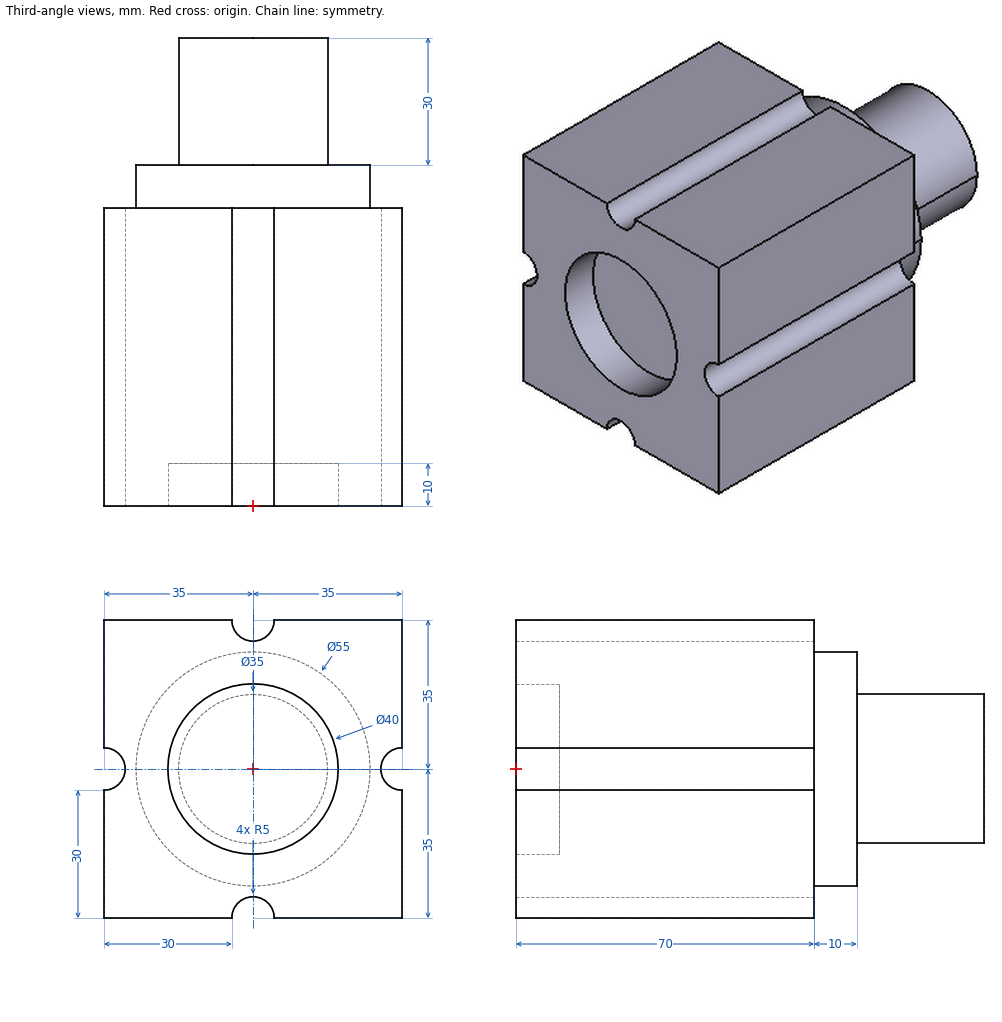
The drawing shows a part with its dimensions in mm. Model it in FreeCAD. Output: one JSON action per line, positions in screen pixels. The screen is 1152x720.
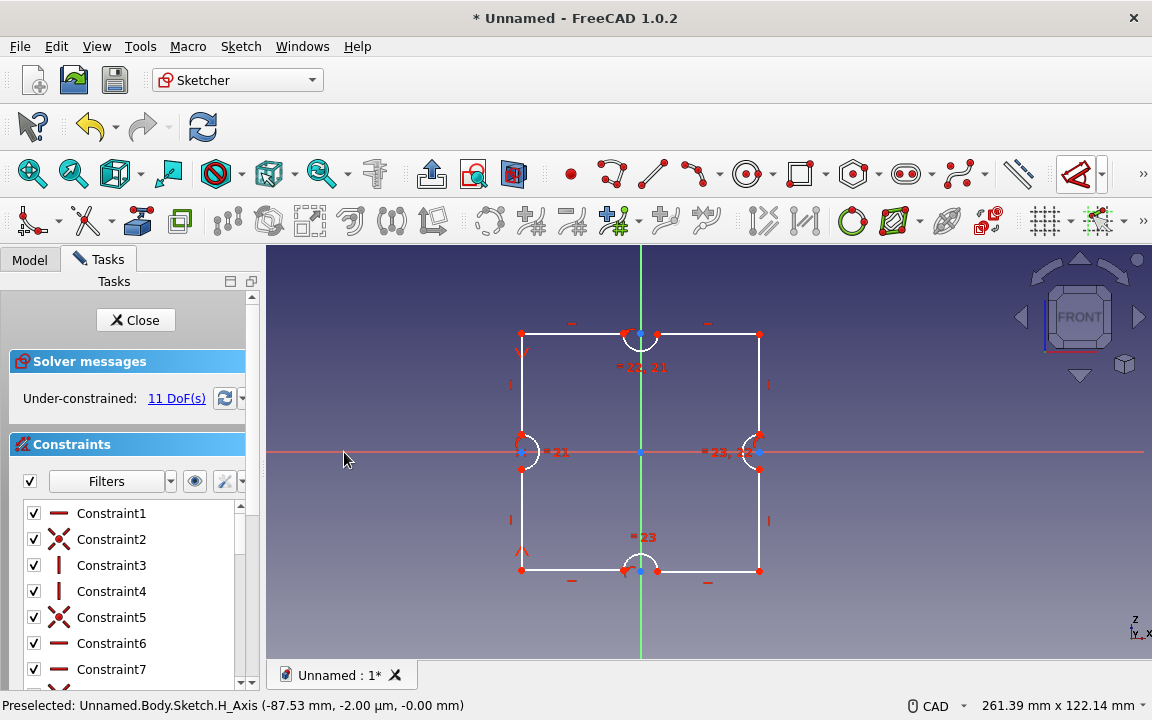
{"action": "left_click", "coordinate": [522, 334]}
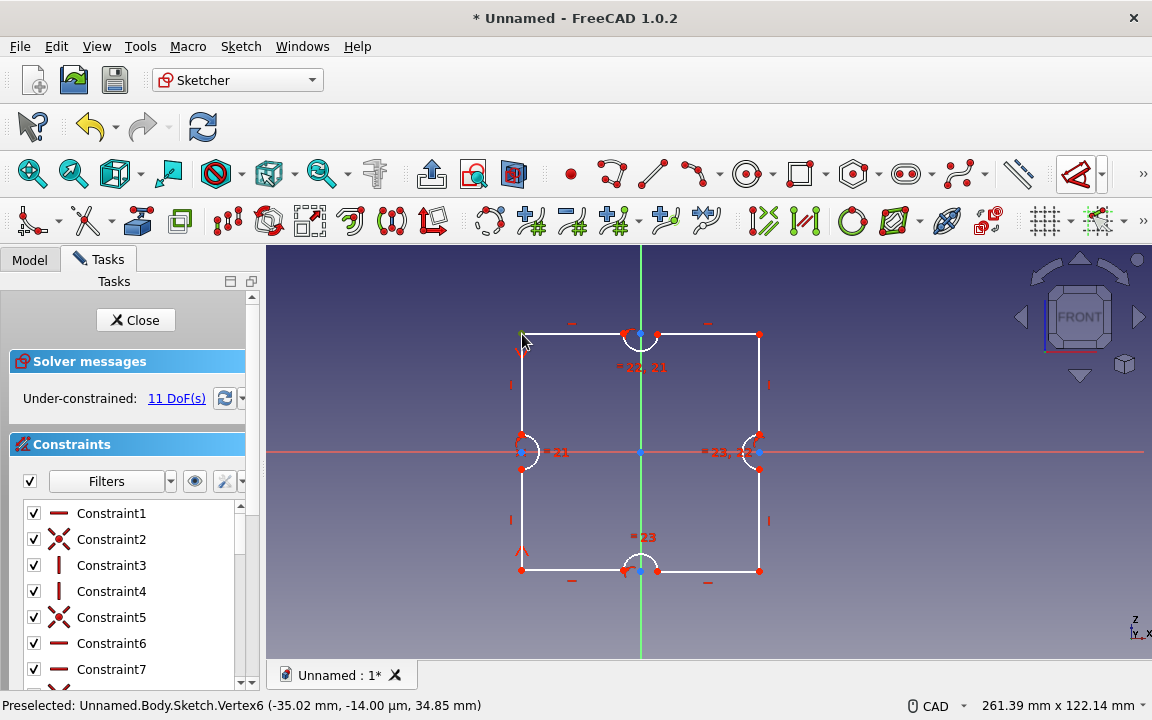
{"action": "left_click", "coordinate": [759, 334]}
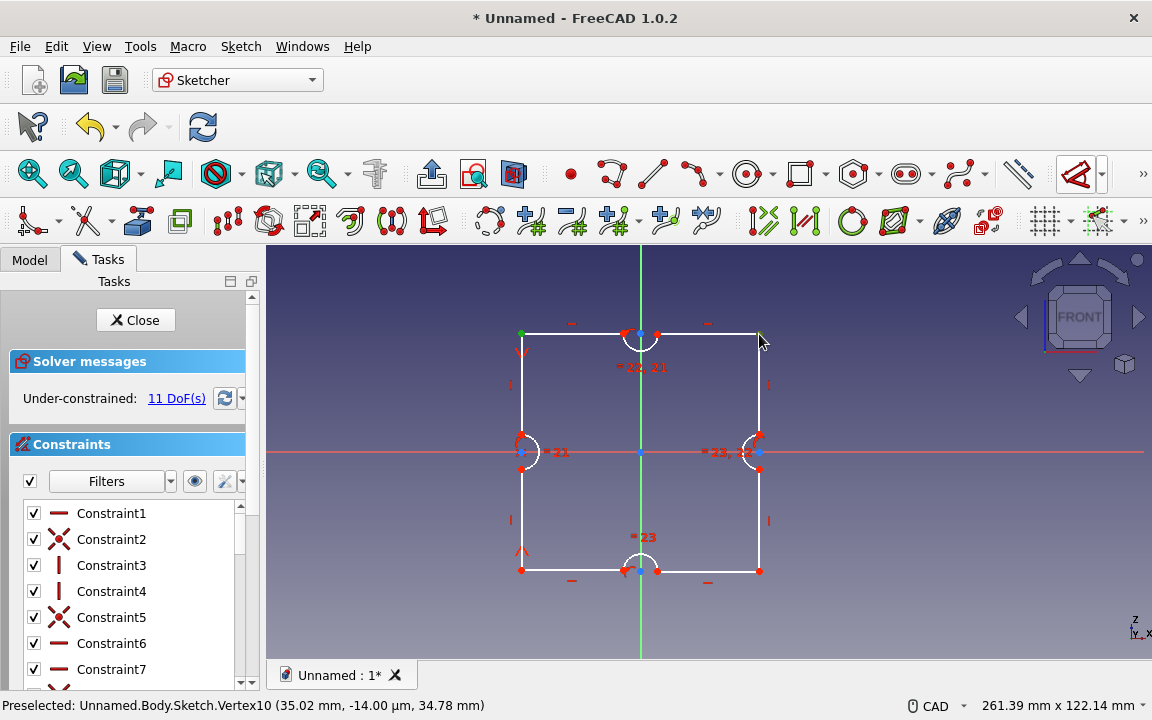
{"action": "left_click", "coordinate": [641, 605]}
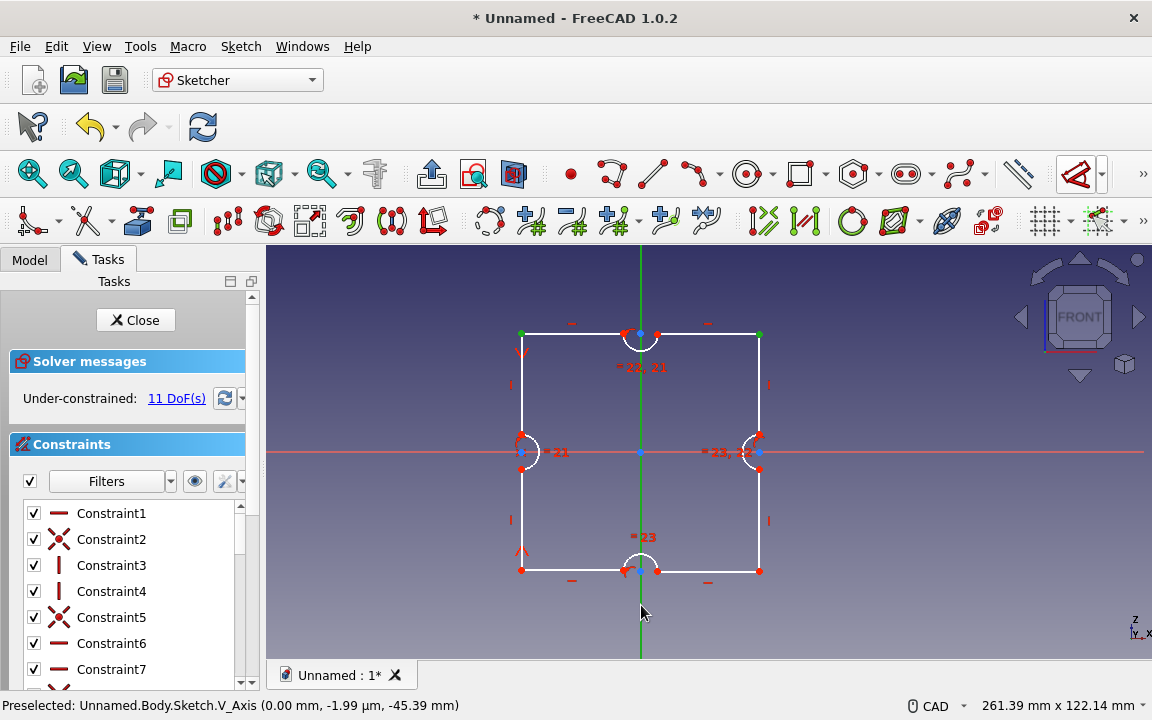
{"action": "key", "text": "s"}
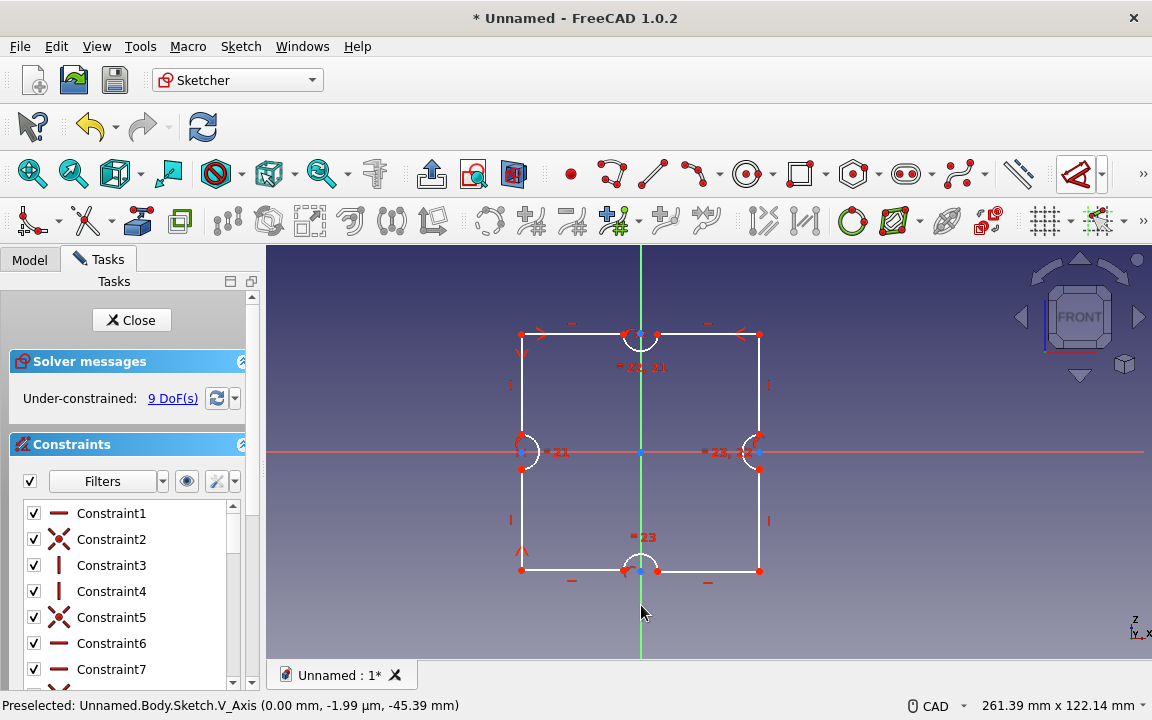
{"action": "left_click", "coordinate": [522, 570]}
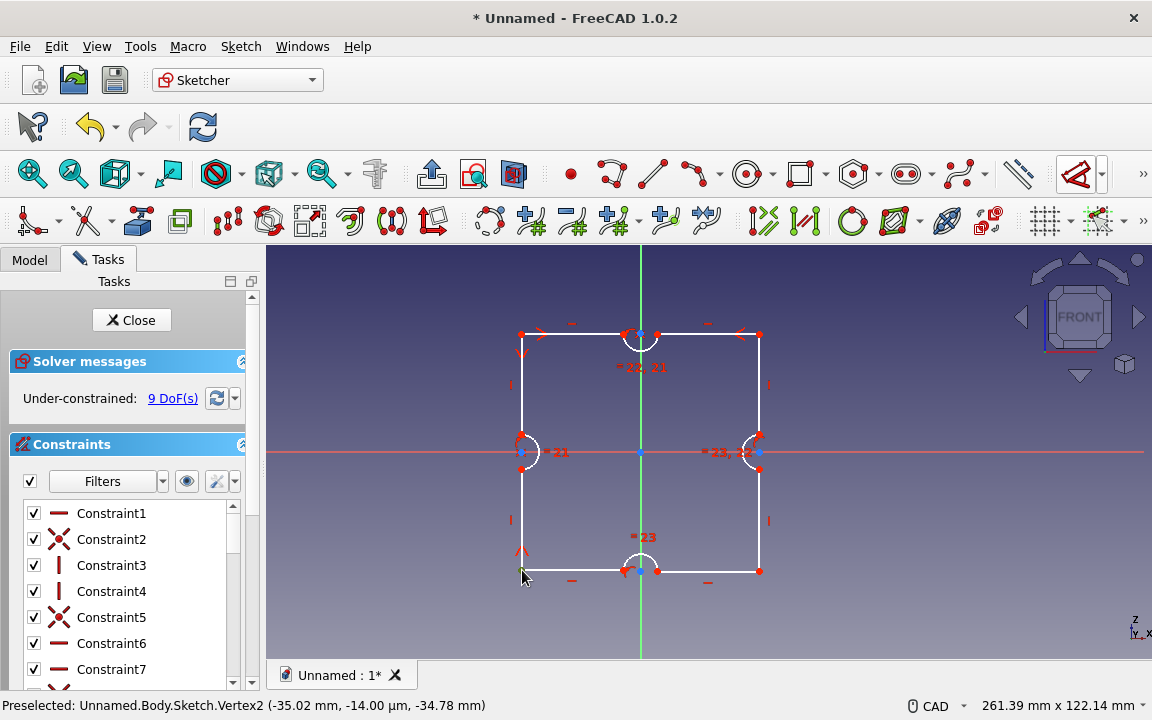
{"action": "left_click", "coordinate": [759, 572]}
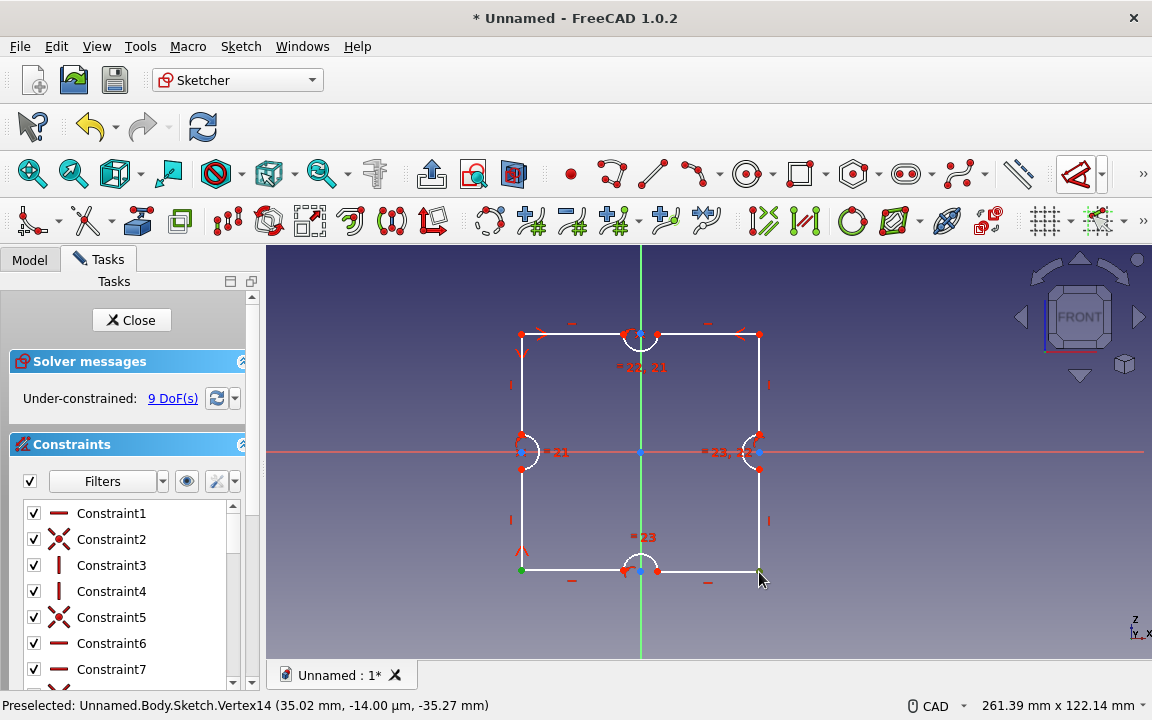
{"action": "left_click", "coordinate": [641, 605]}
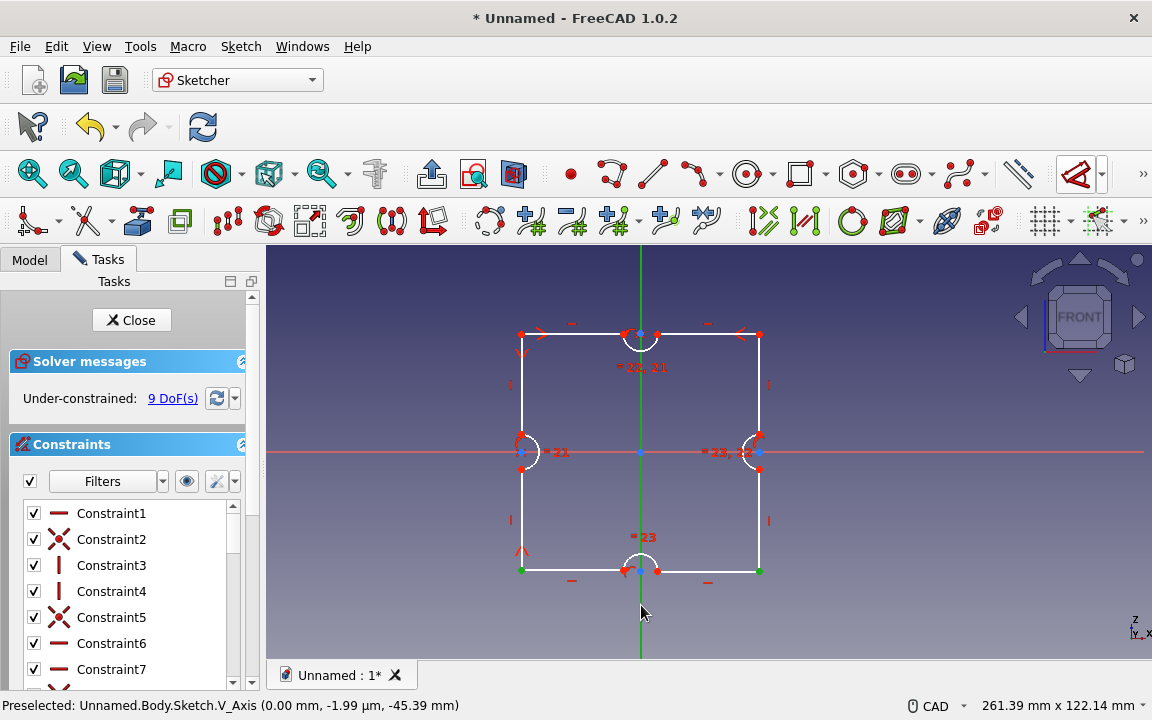
{"action": "key", "text": "s"}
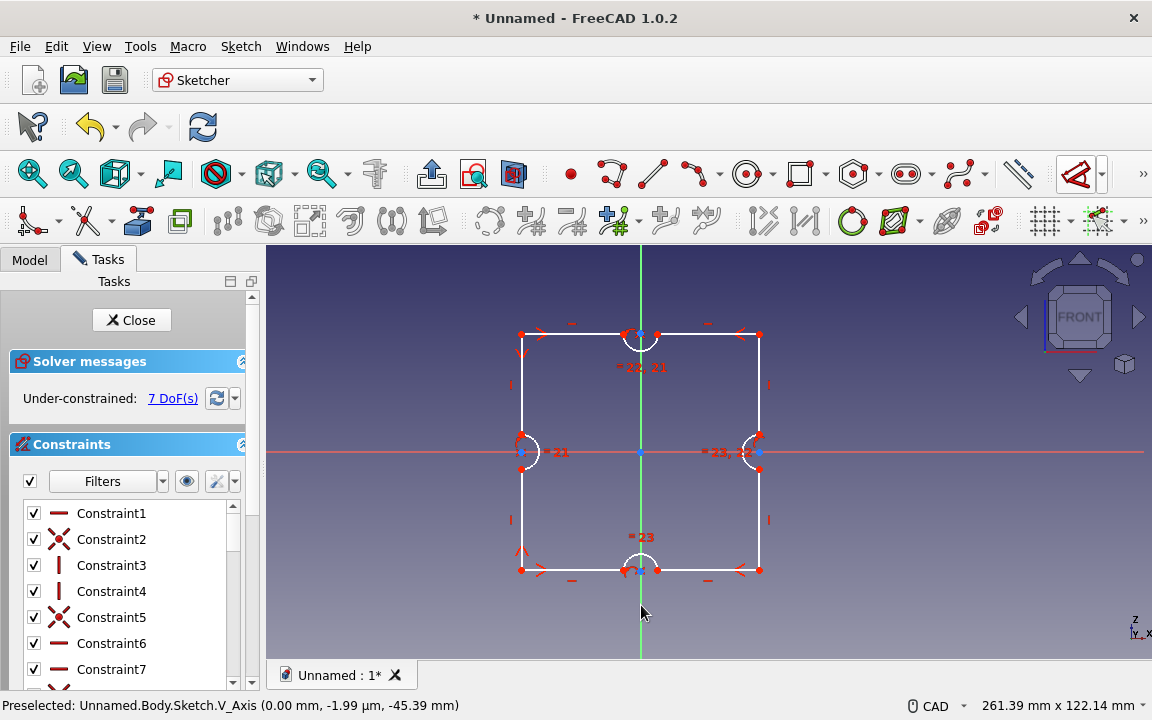
{"action": "scroll", "coordinate": [536, 462], "scroll_direction": "up", "scroll_amount": 5}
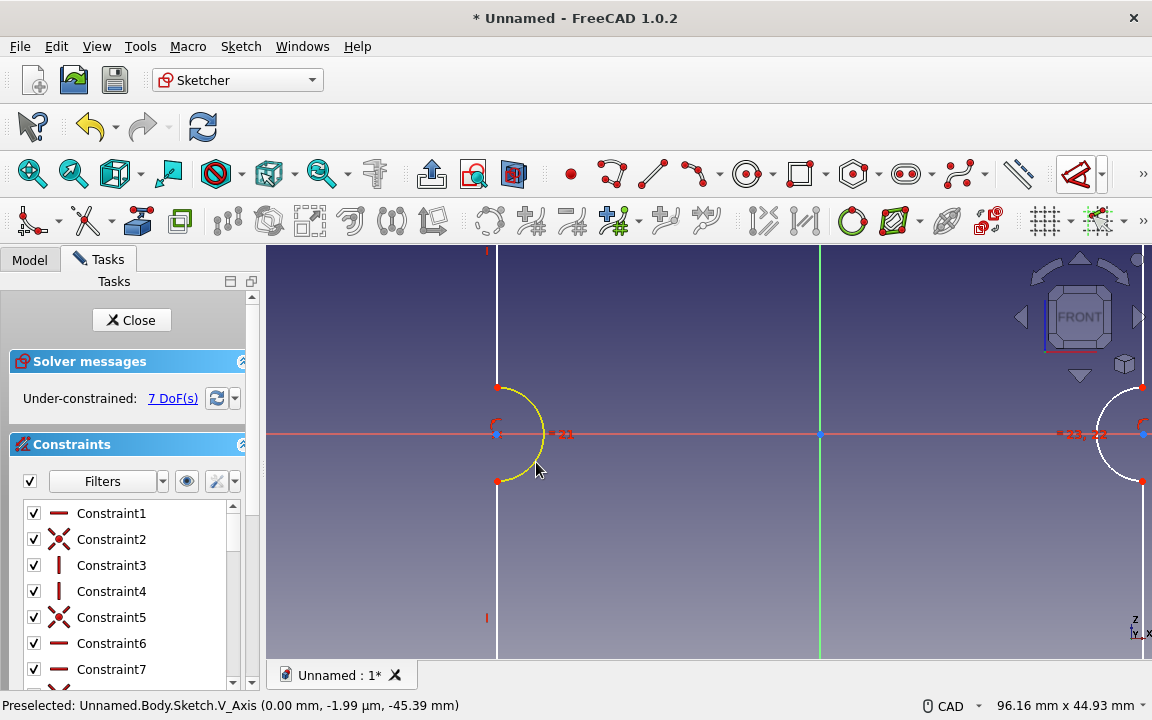
{"action": "left_click", "coordinate": [535, 462]}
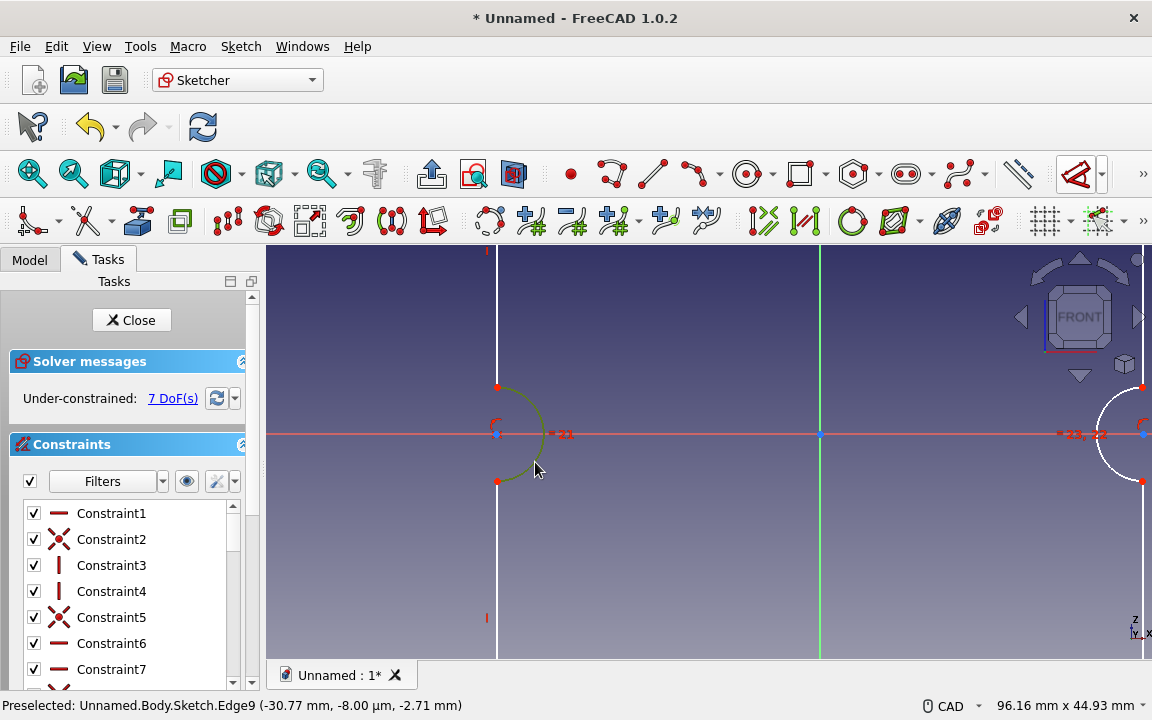
{"action": "key", "text": "k r"}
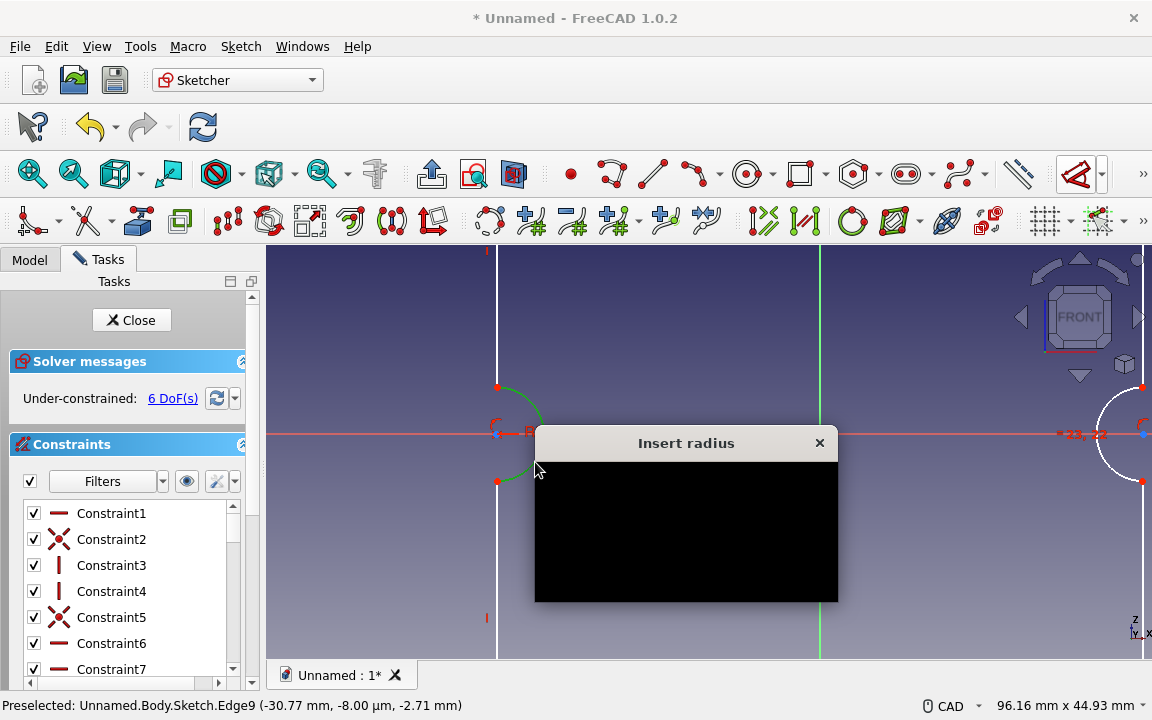
{"action": "type", "text": "5"}
{"action": "key", "text": "Return"}